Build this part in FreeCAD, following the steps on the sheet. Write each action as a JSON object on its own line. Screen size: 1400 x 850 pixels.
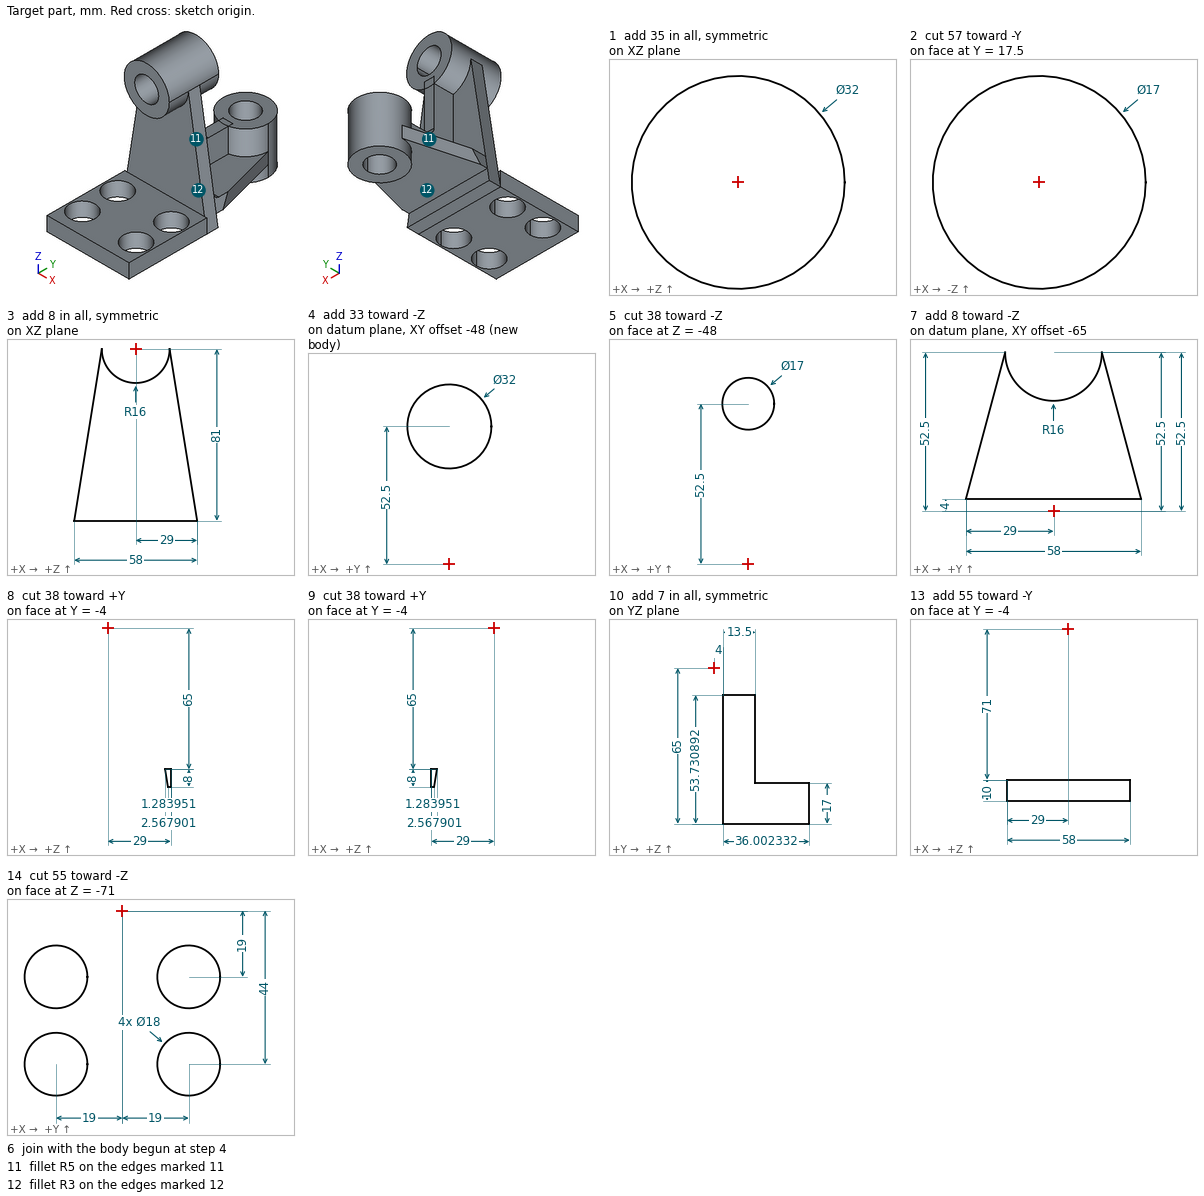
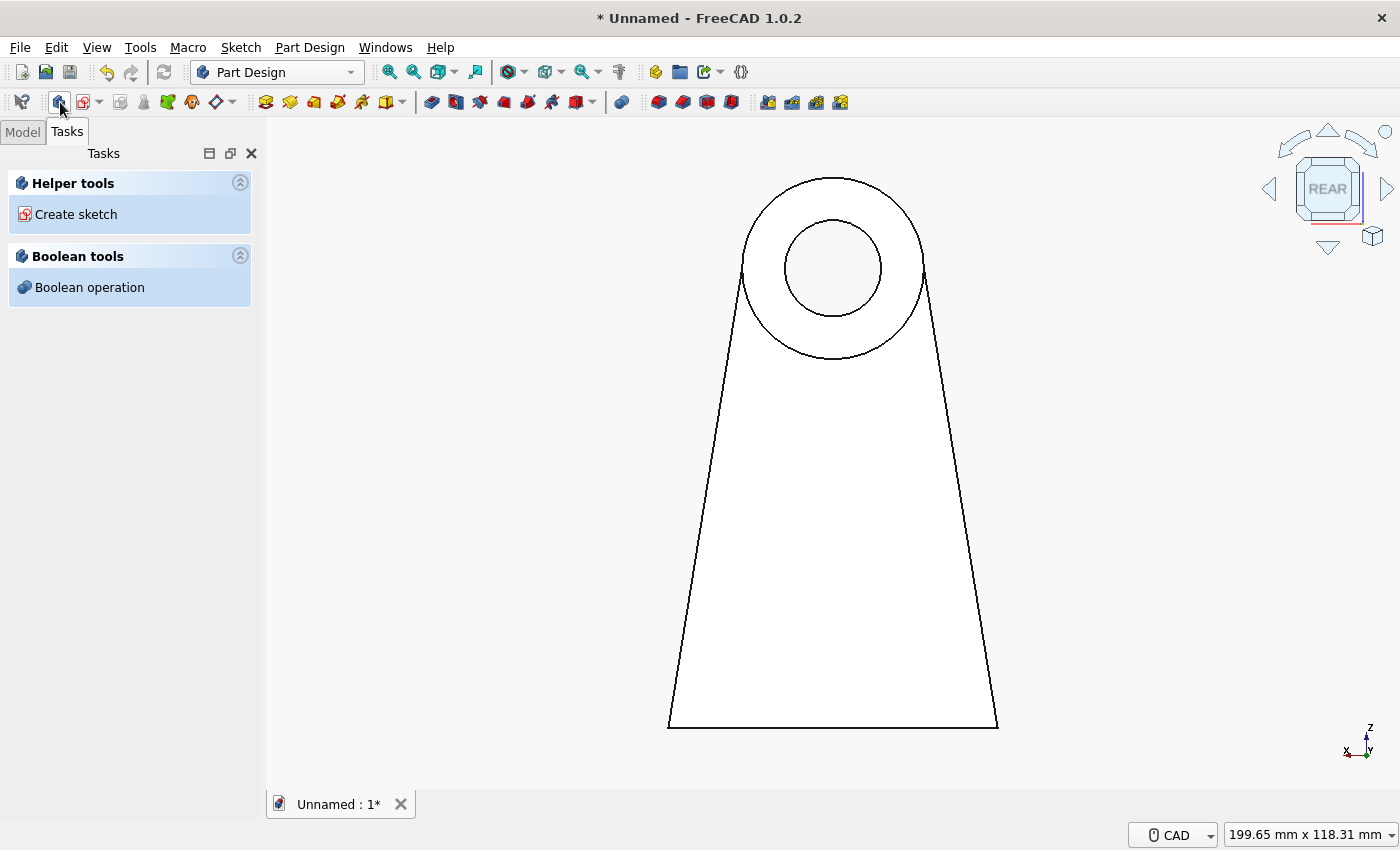
{"action": "left_click", "coordinate": [23, 131]}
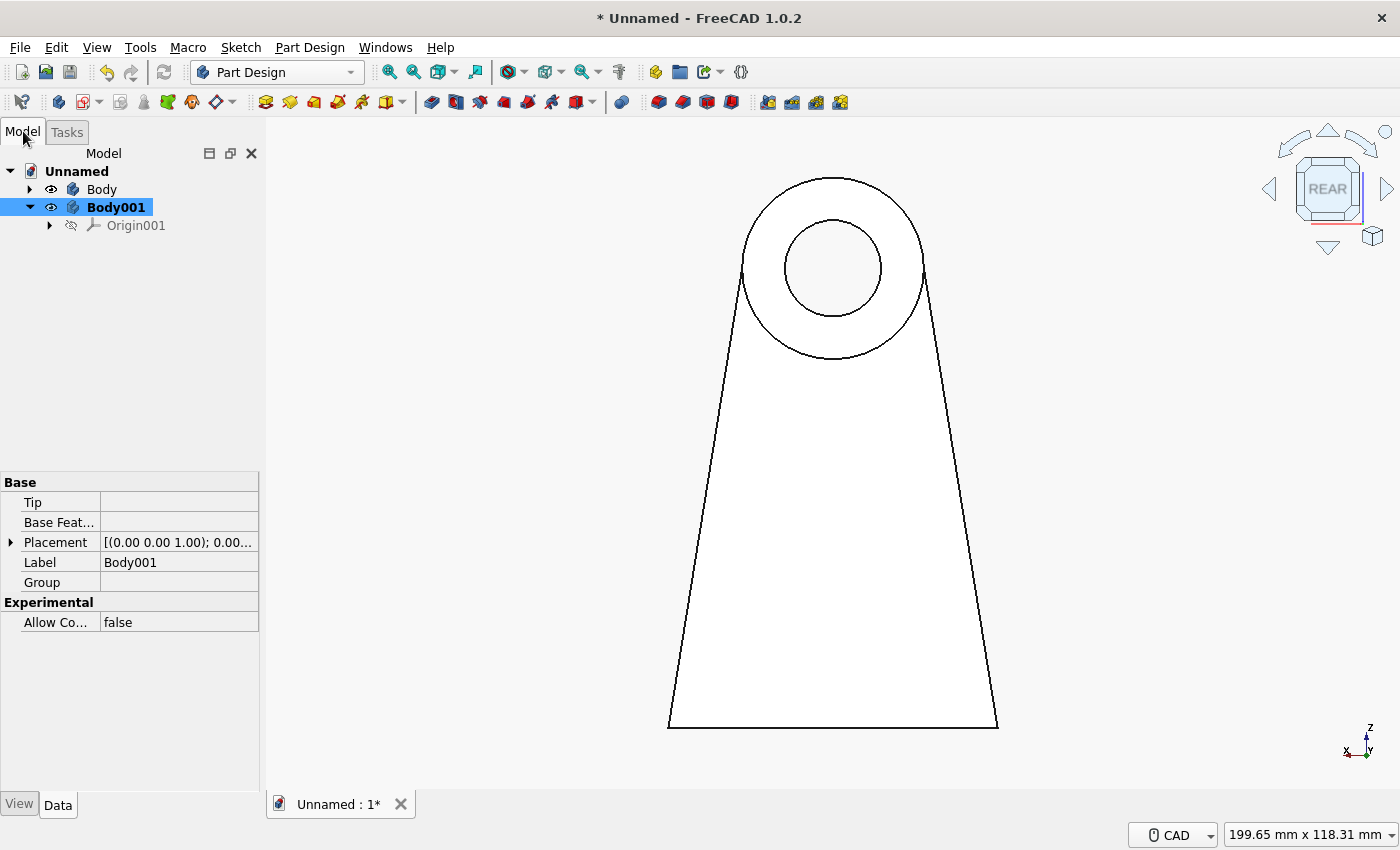
{"action": "left_click", "coordinate": [50, 225]}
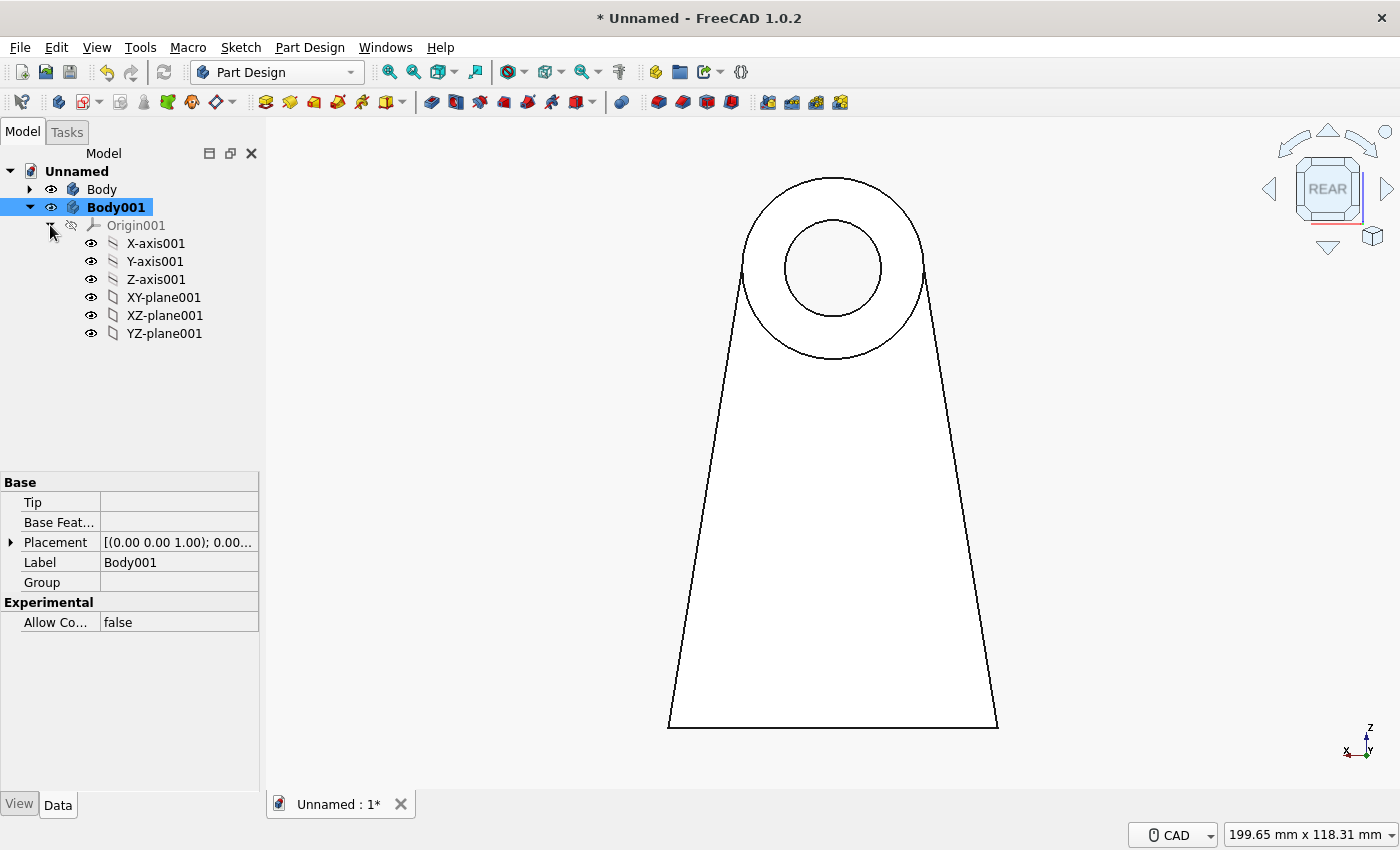
{"action": "left_click", "coordinate": [136, 297]}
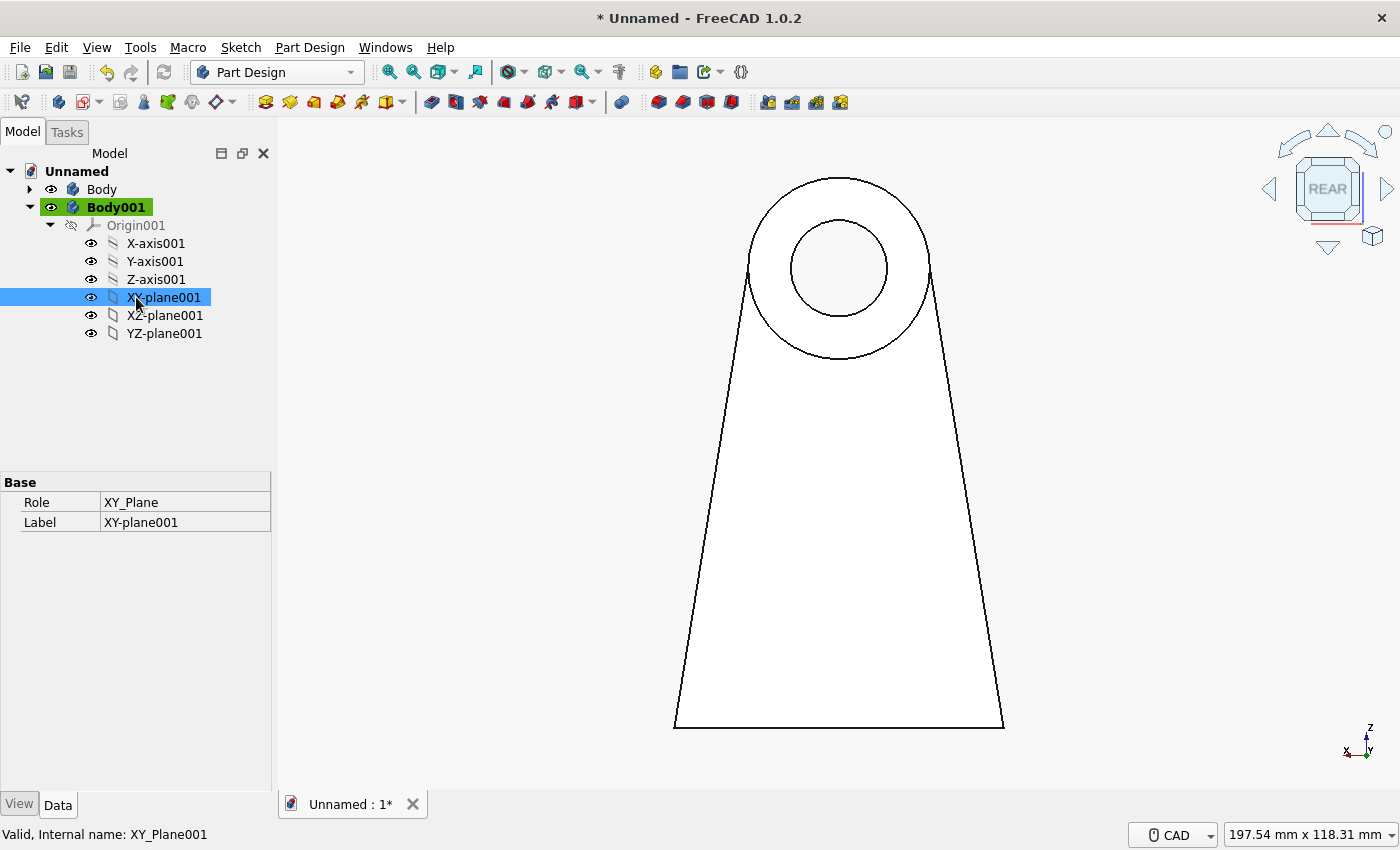
{"action": "left_click", "coordinate": [216, 102]}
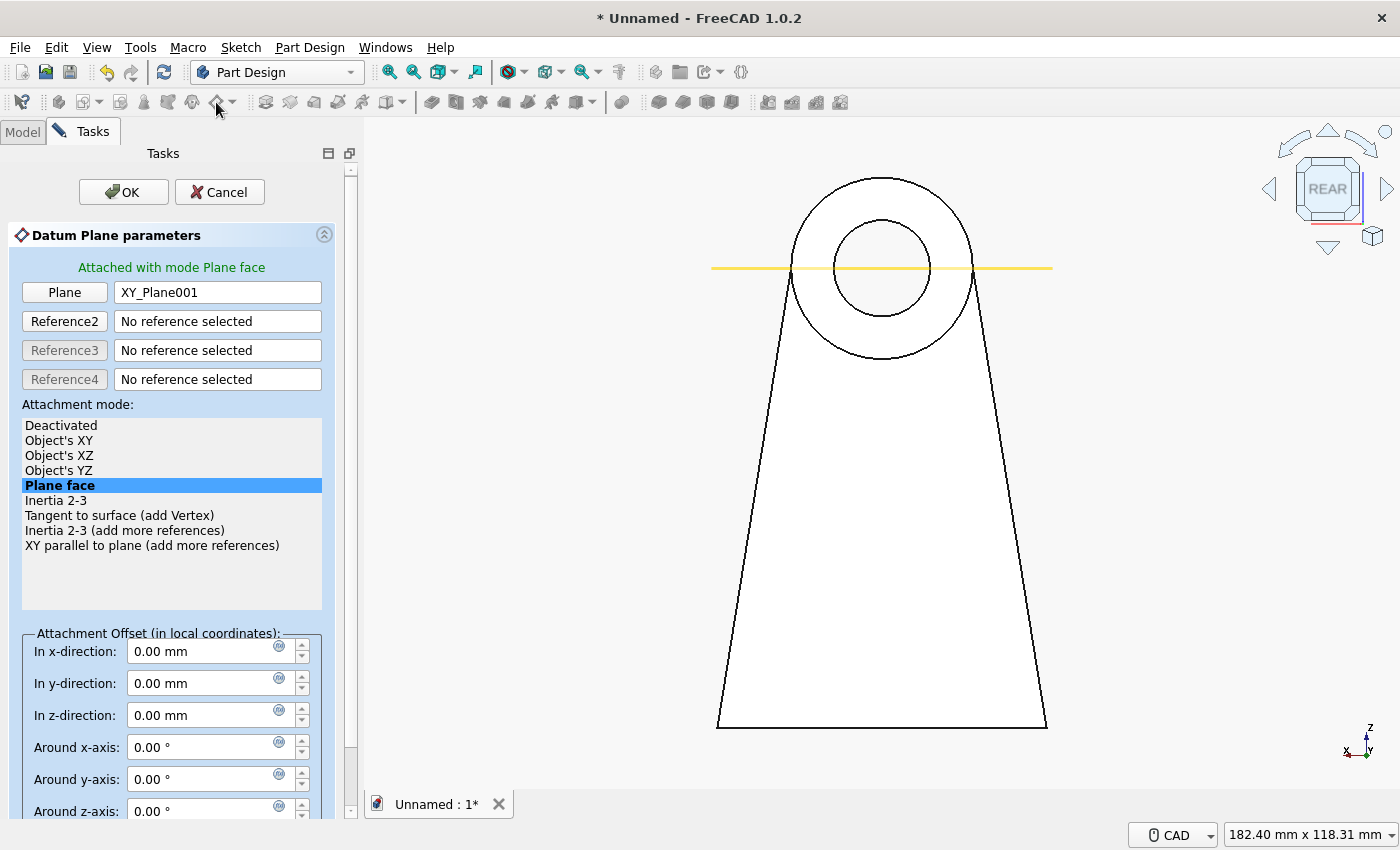
{"action": "triple_click", "coordinate": [210, 715]}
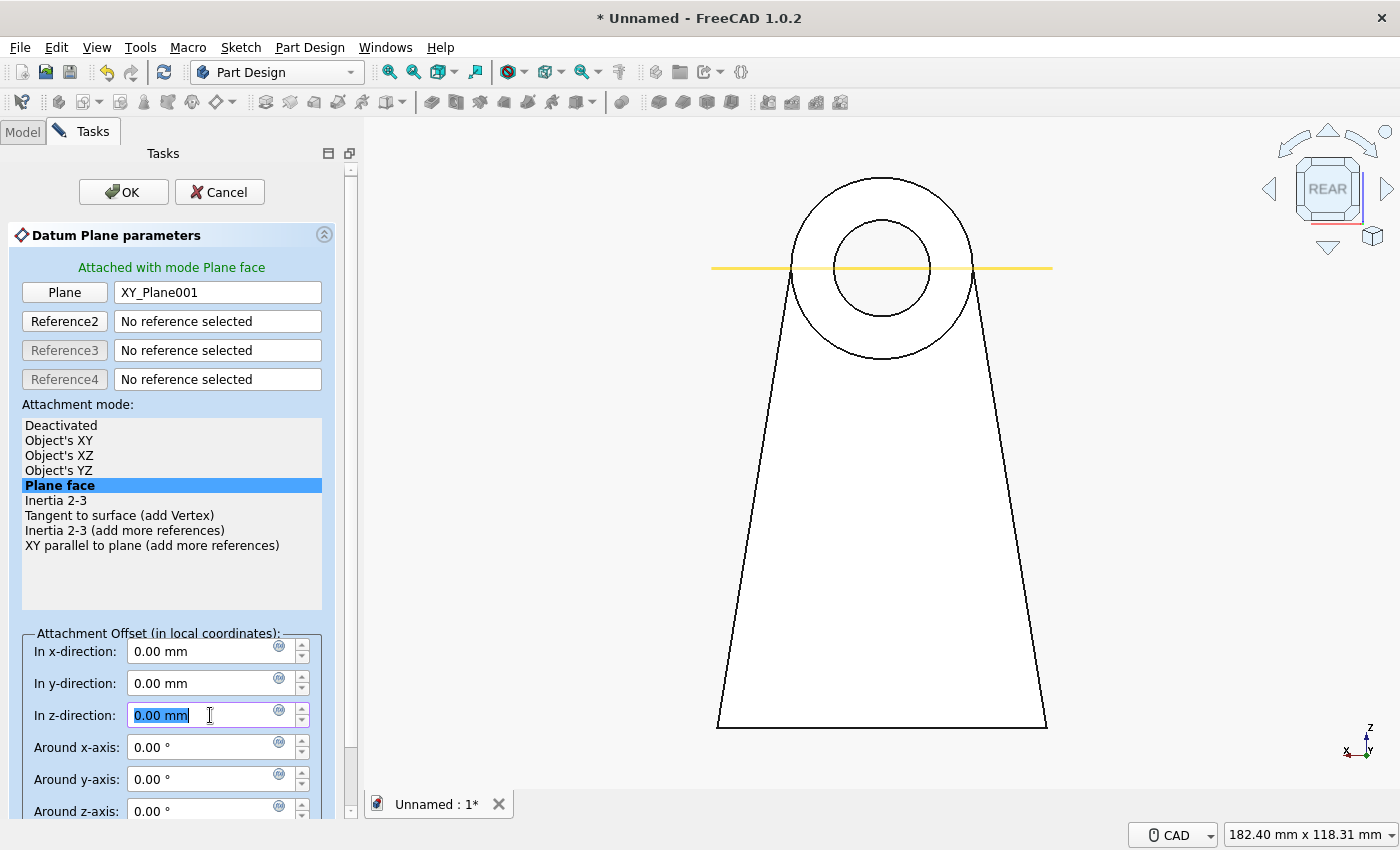
{"action": "type", "text": "-48"}
{"action": "key", "text": "Tab"}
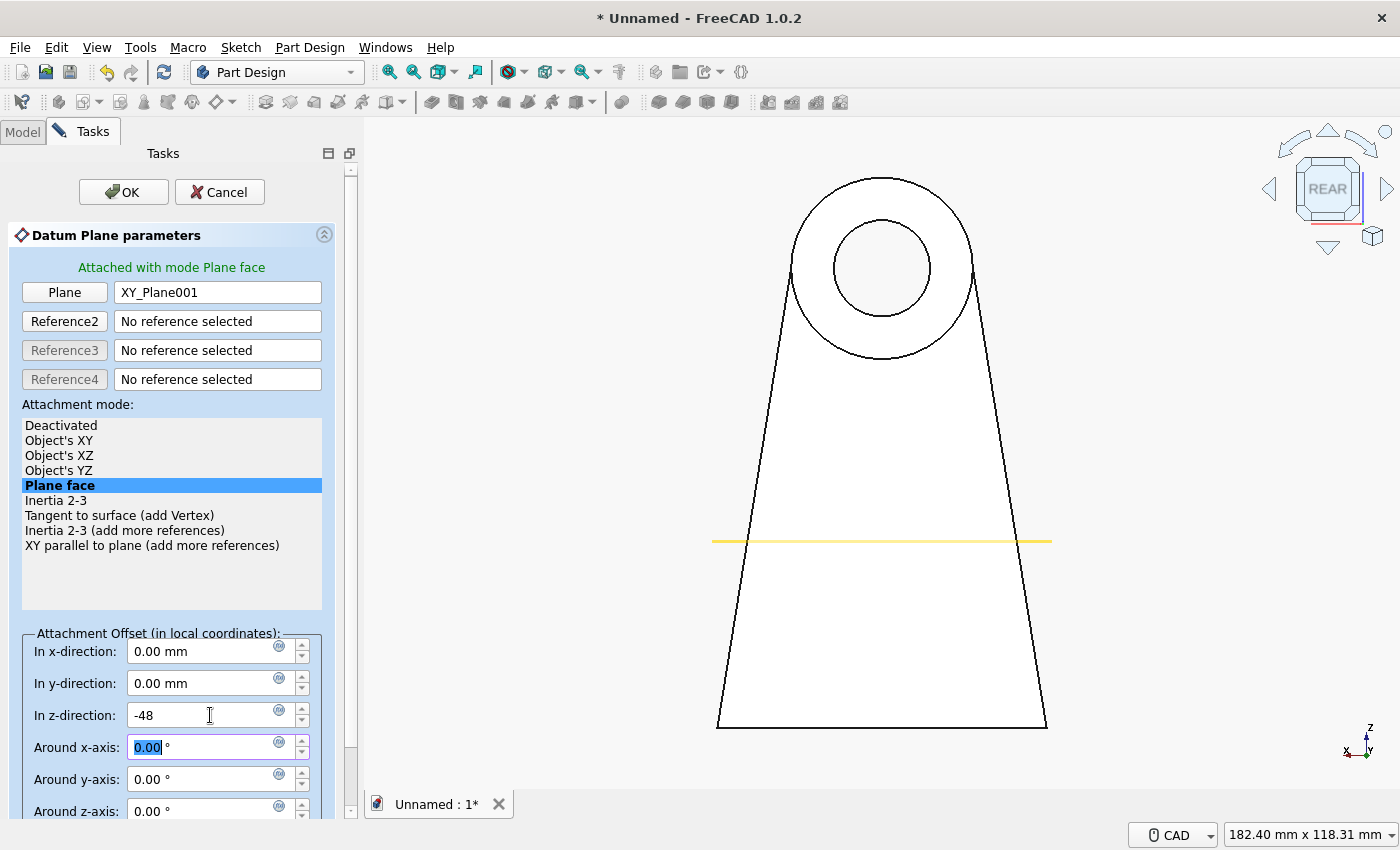
{"action": "left_click", "coordinate": [124, 192]}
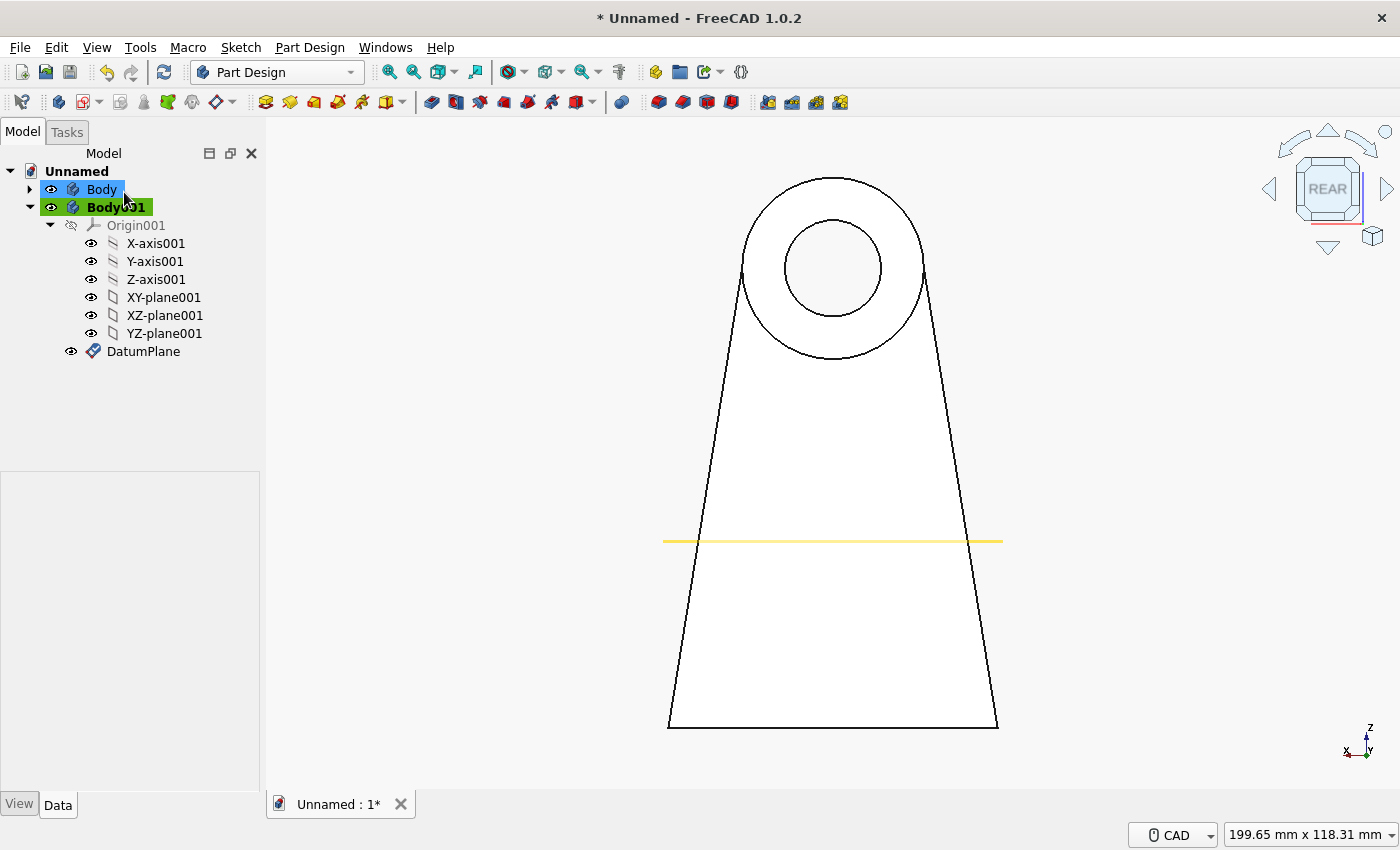
{"action": "left_click", "coordinate": [116, 351]}